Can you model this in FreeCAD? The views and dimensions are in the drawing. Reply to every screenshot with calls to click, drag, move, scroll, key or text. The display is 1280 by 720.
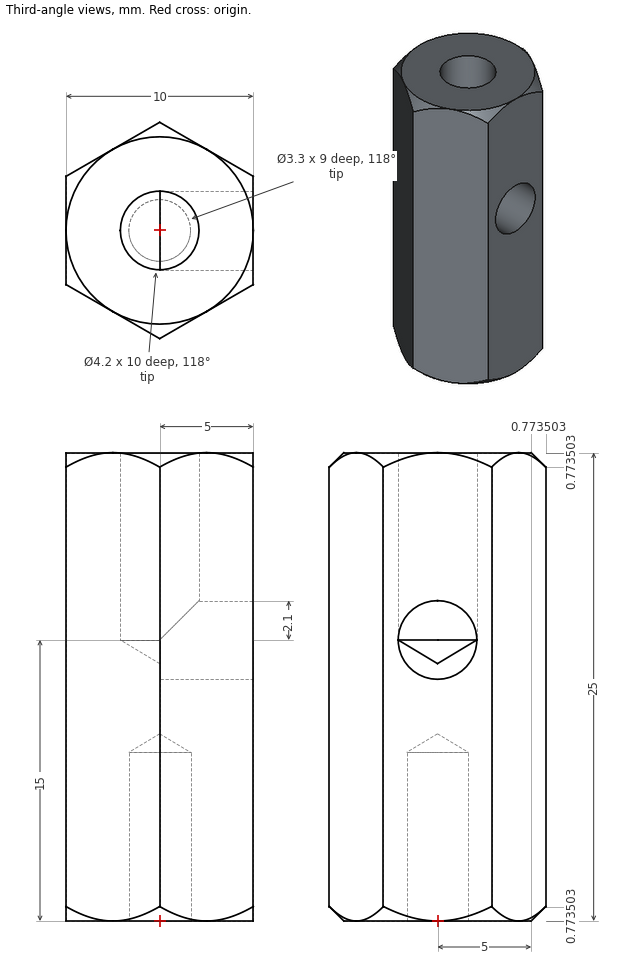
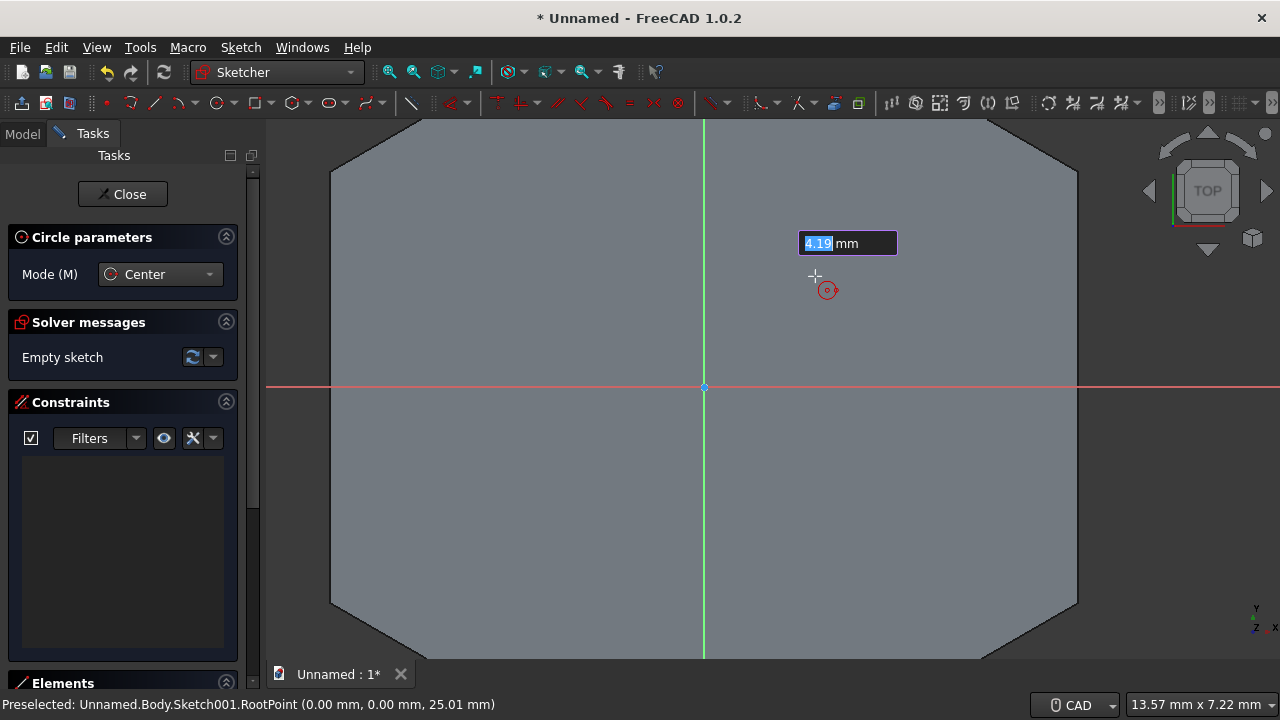
text(4.2)
key(Return)
key(Escape)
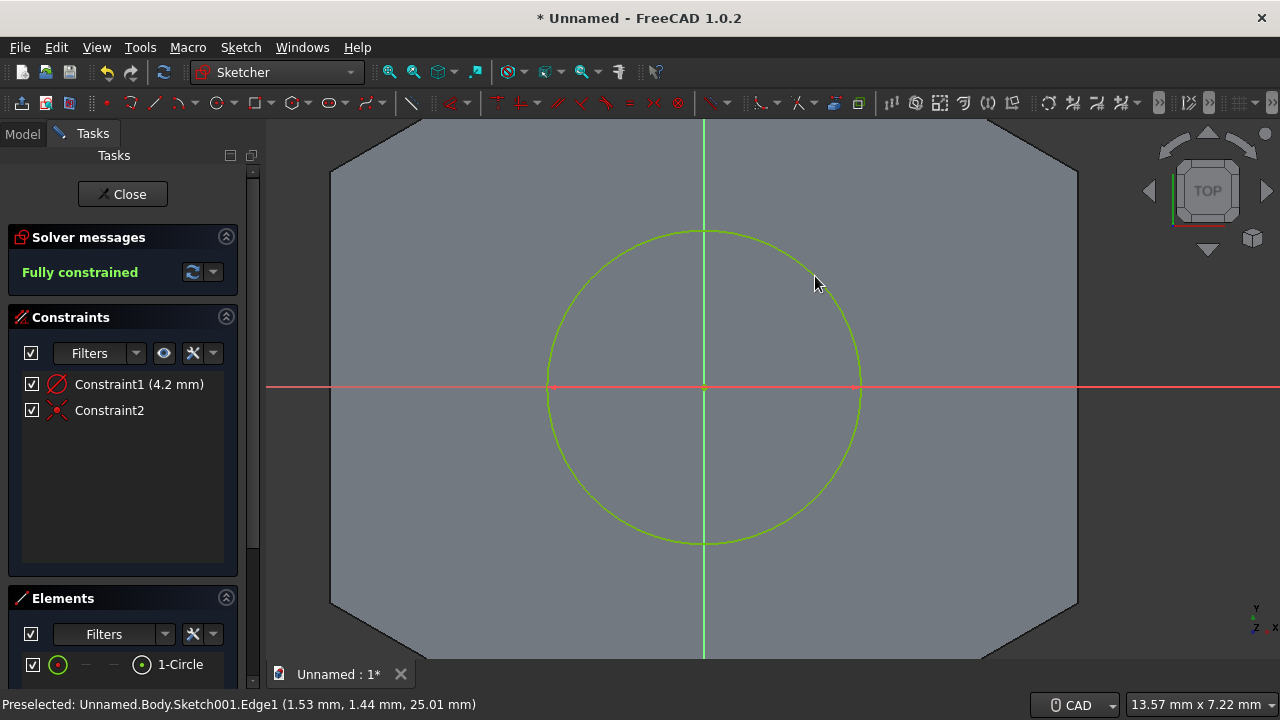
click(123, 194)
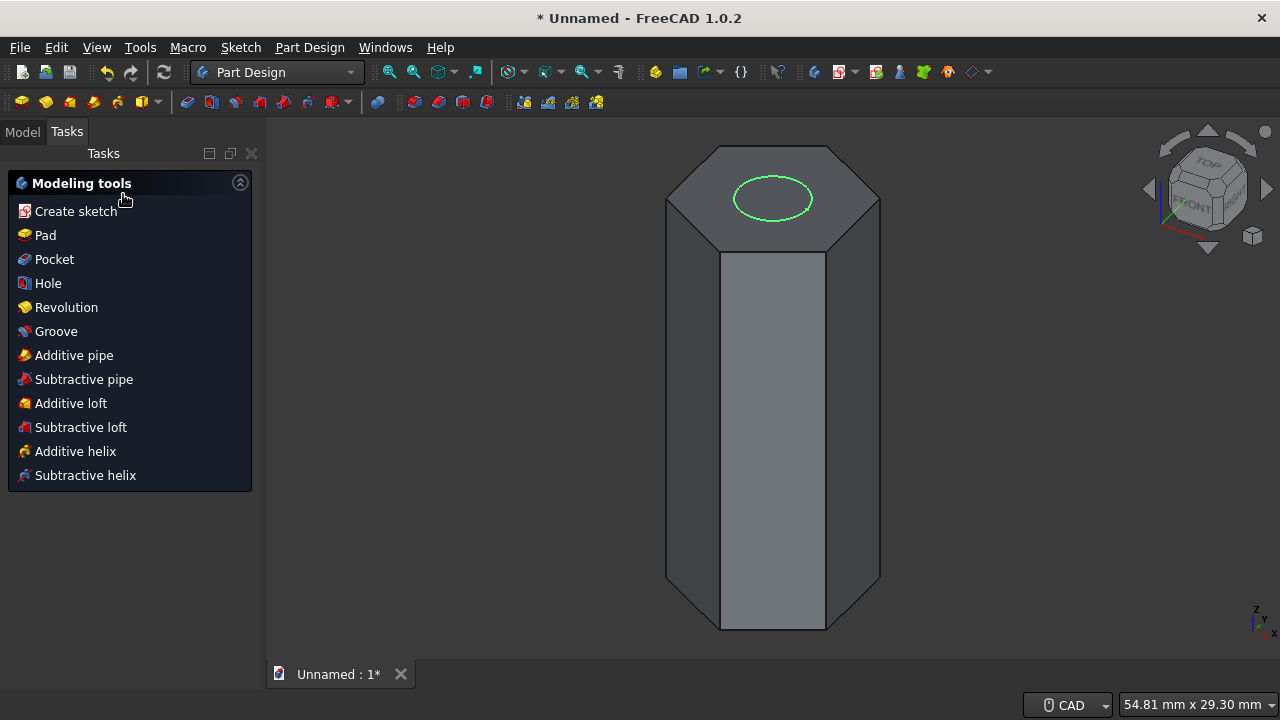
click(212, 102)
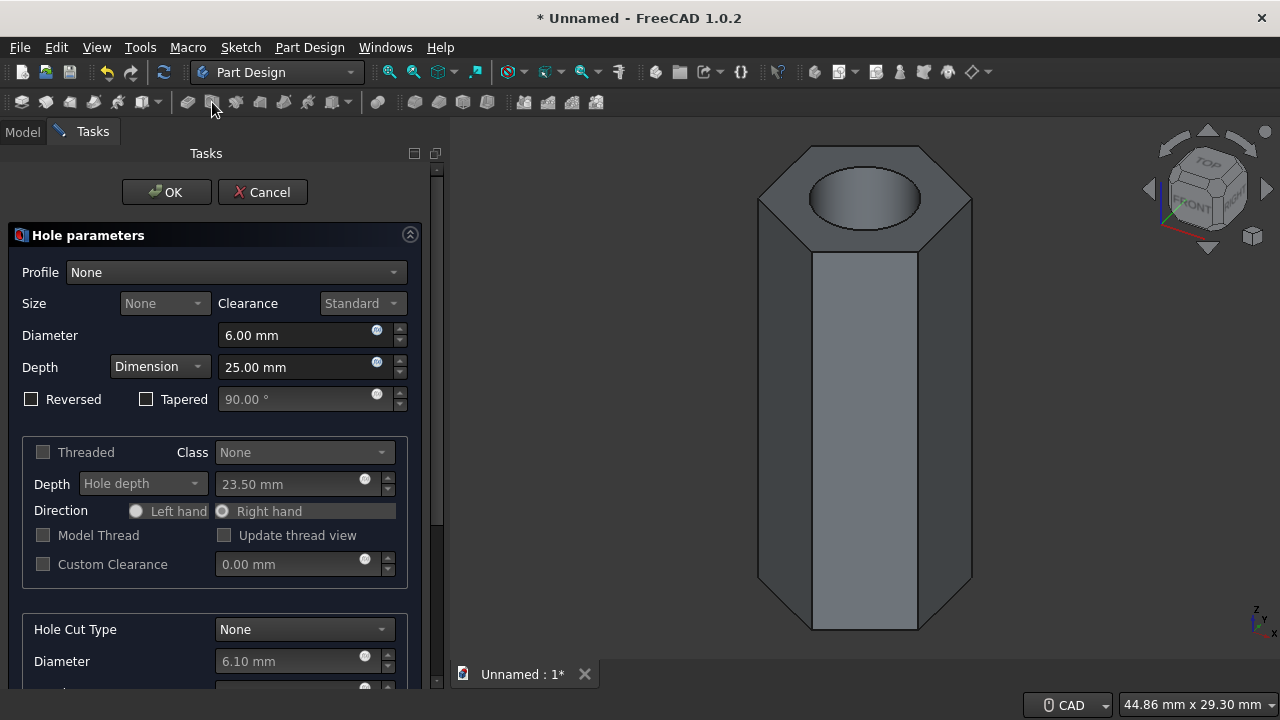
triple_click(305, 335)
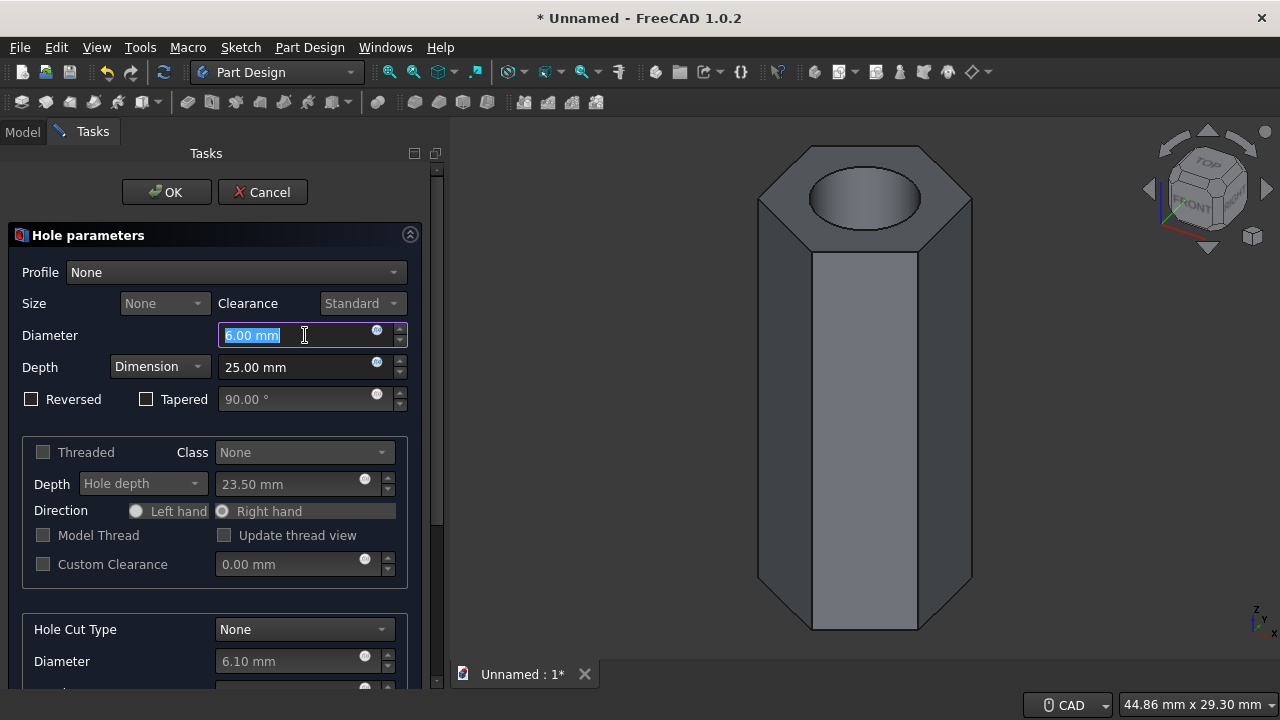
text(4.2)
key(Tab)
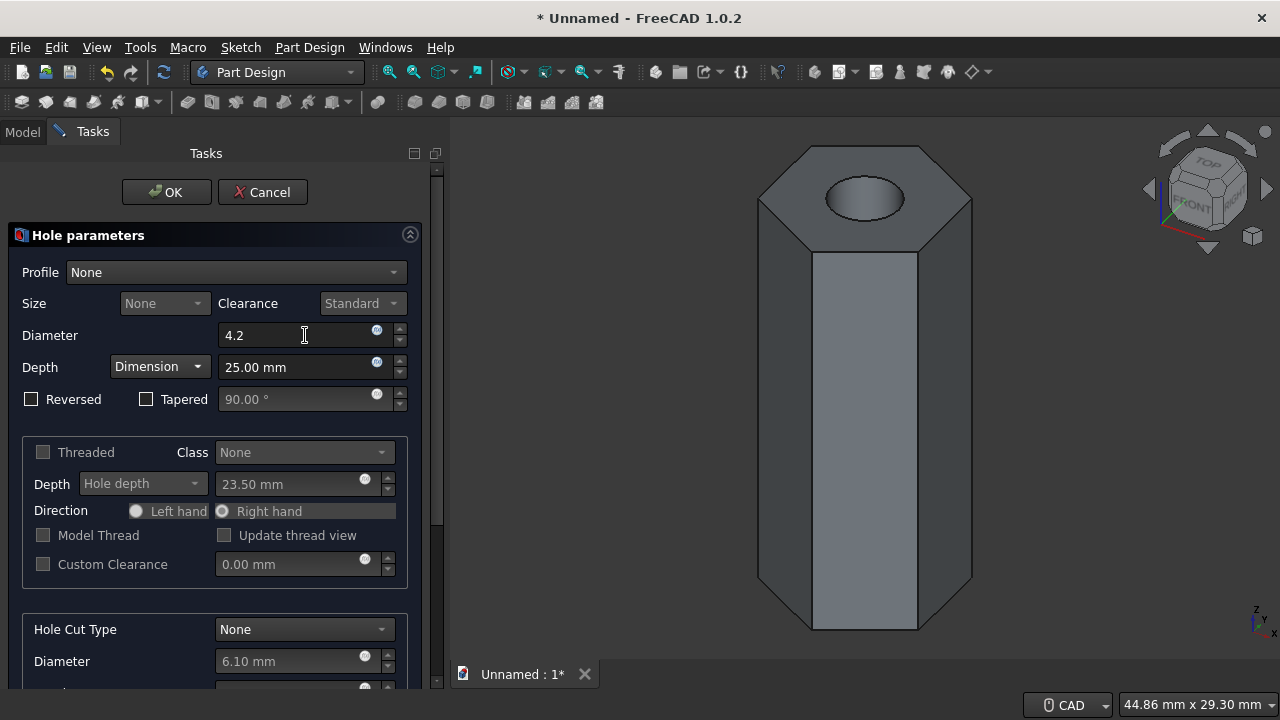
triple_click(305, 367)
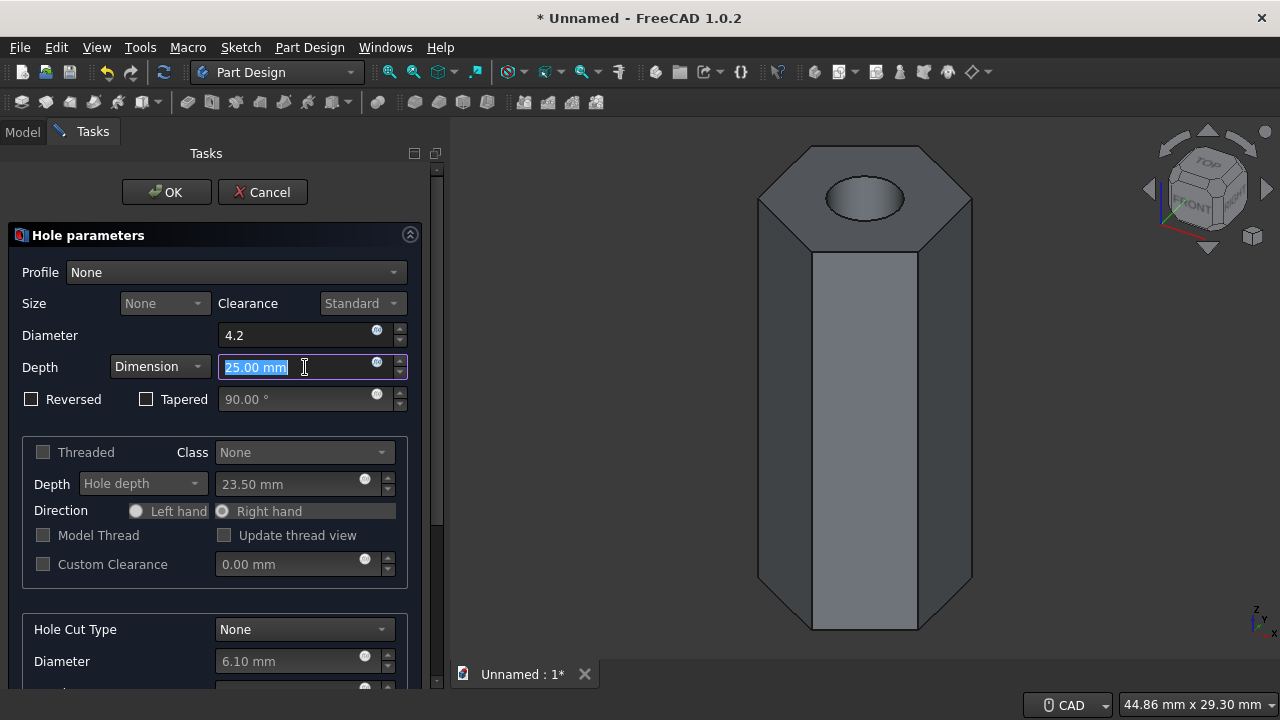
text(10)
key(Tab)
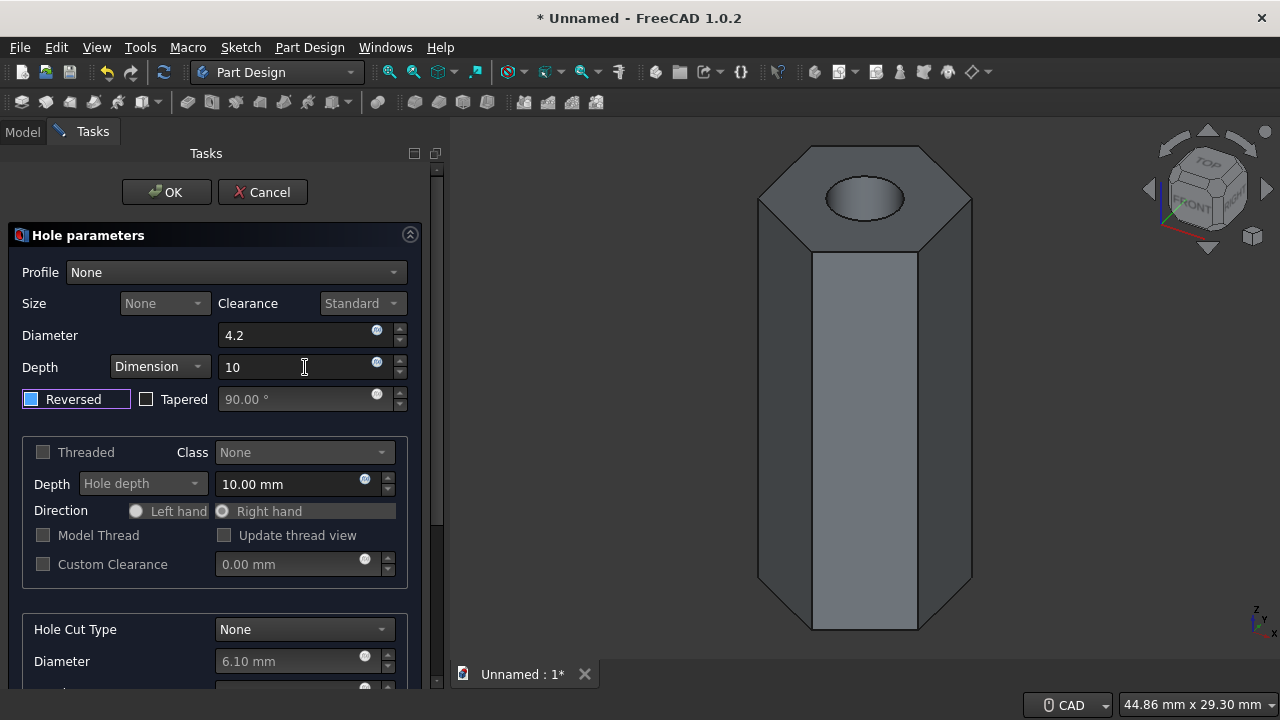
click(167, 192)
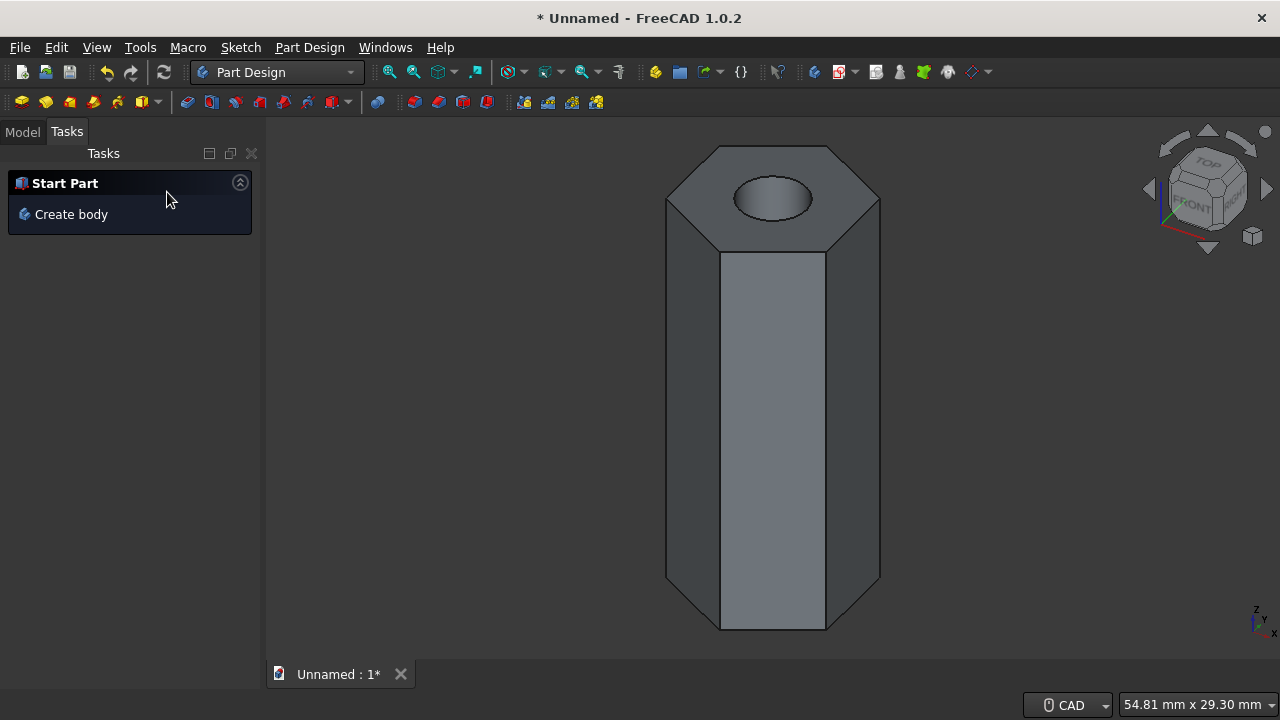
click(840, 72)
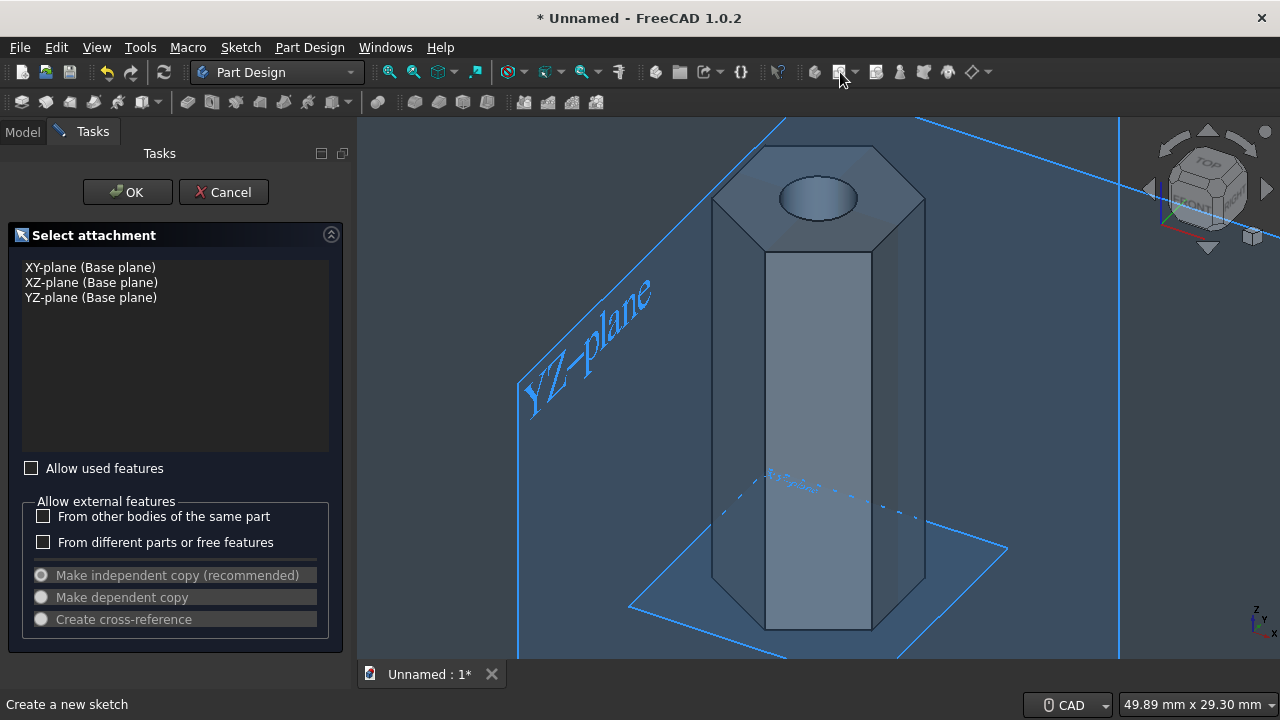
click(82, 268)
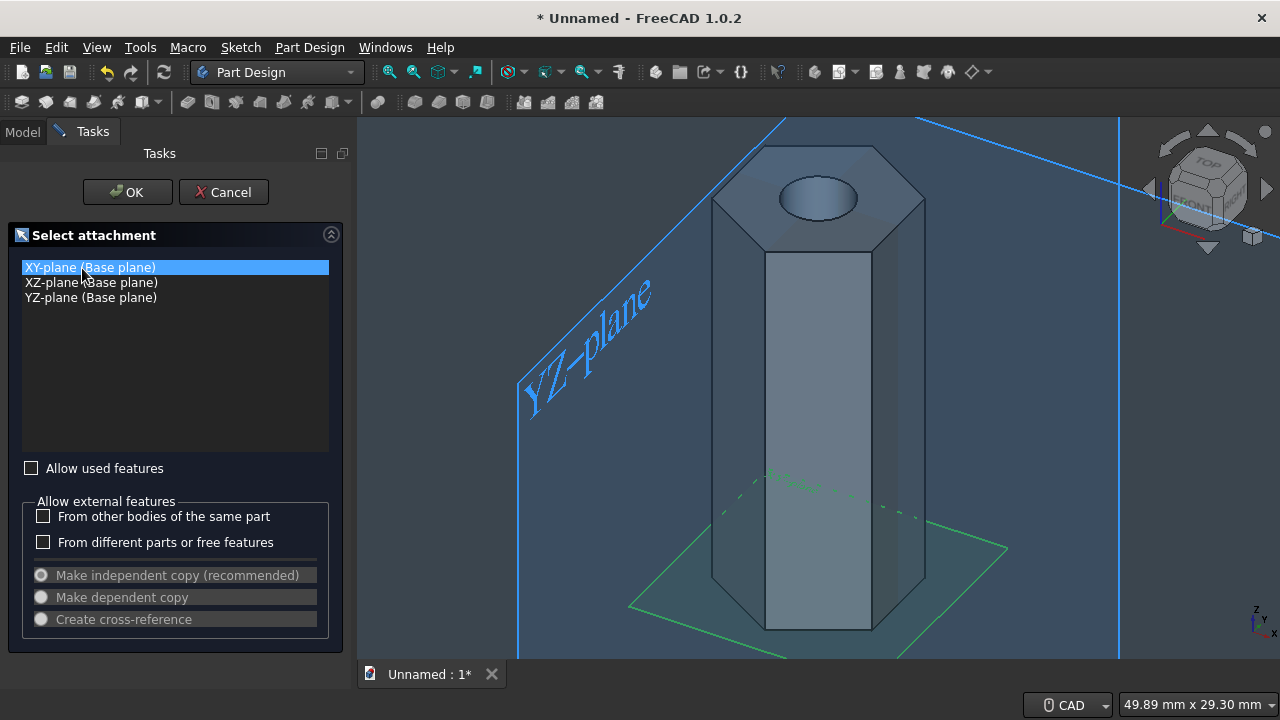
click(128, 192)